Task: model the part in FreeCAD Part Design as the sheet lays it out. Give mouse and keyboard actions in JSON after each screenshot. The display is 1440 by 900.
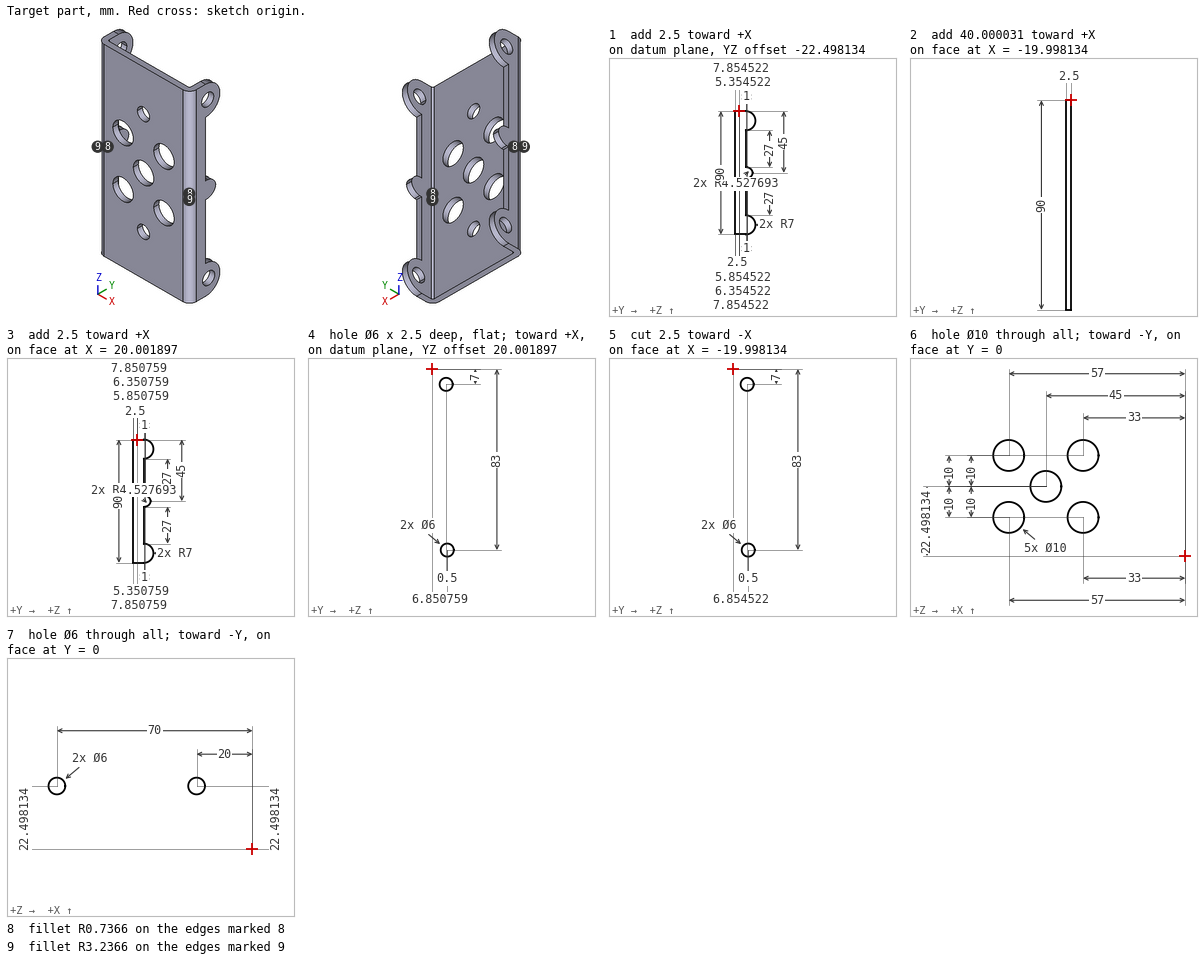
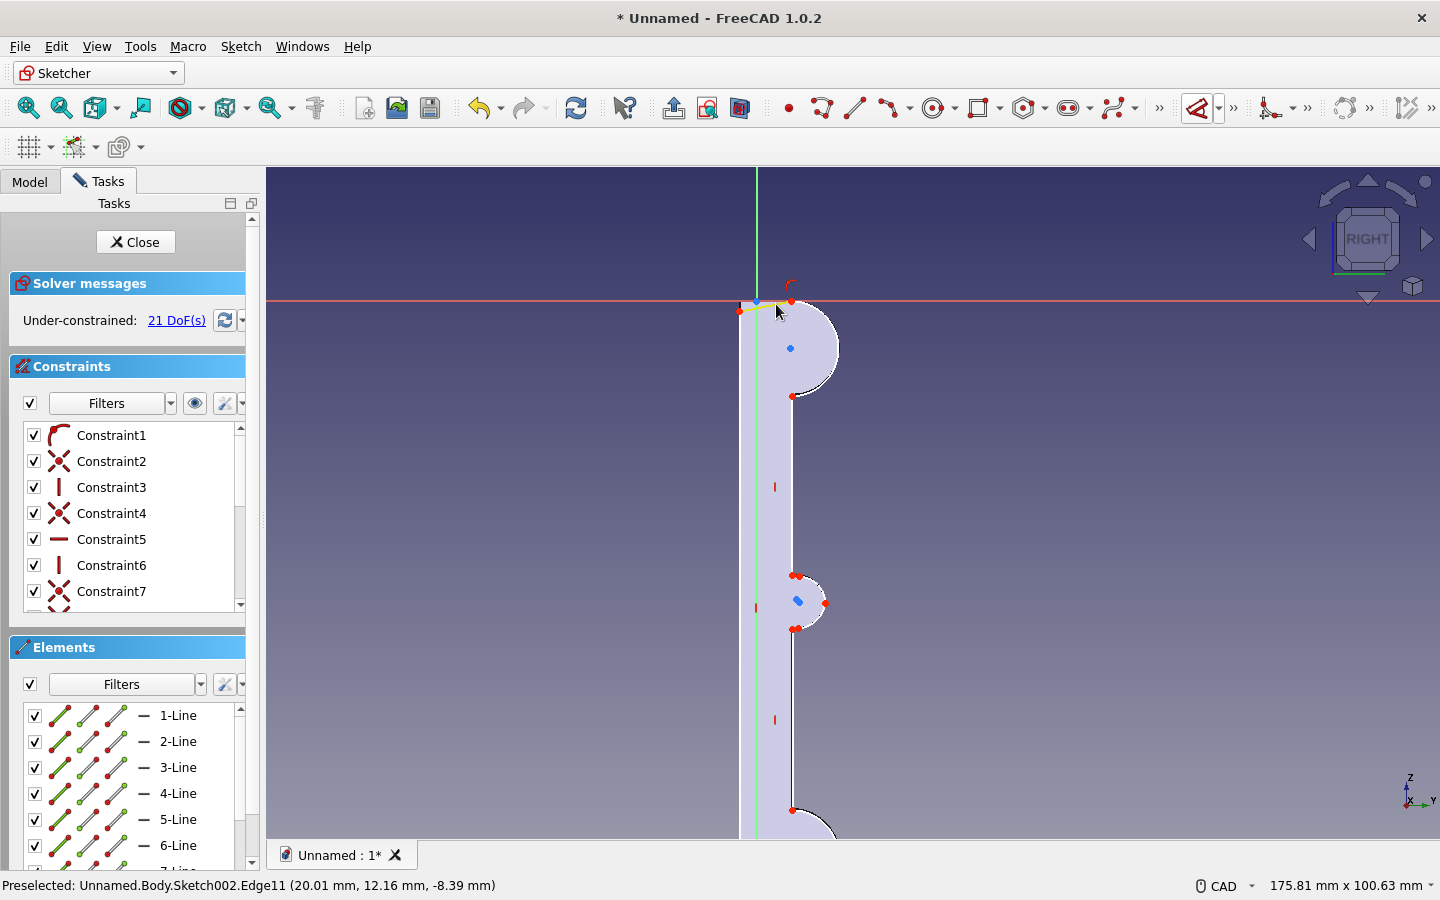
{"action": "left_click", "coordinate": [776, 304]}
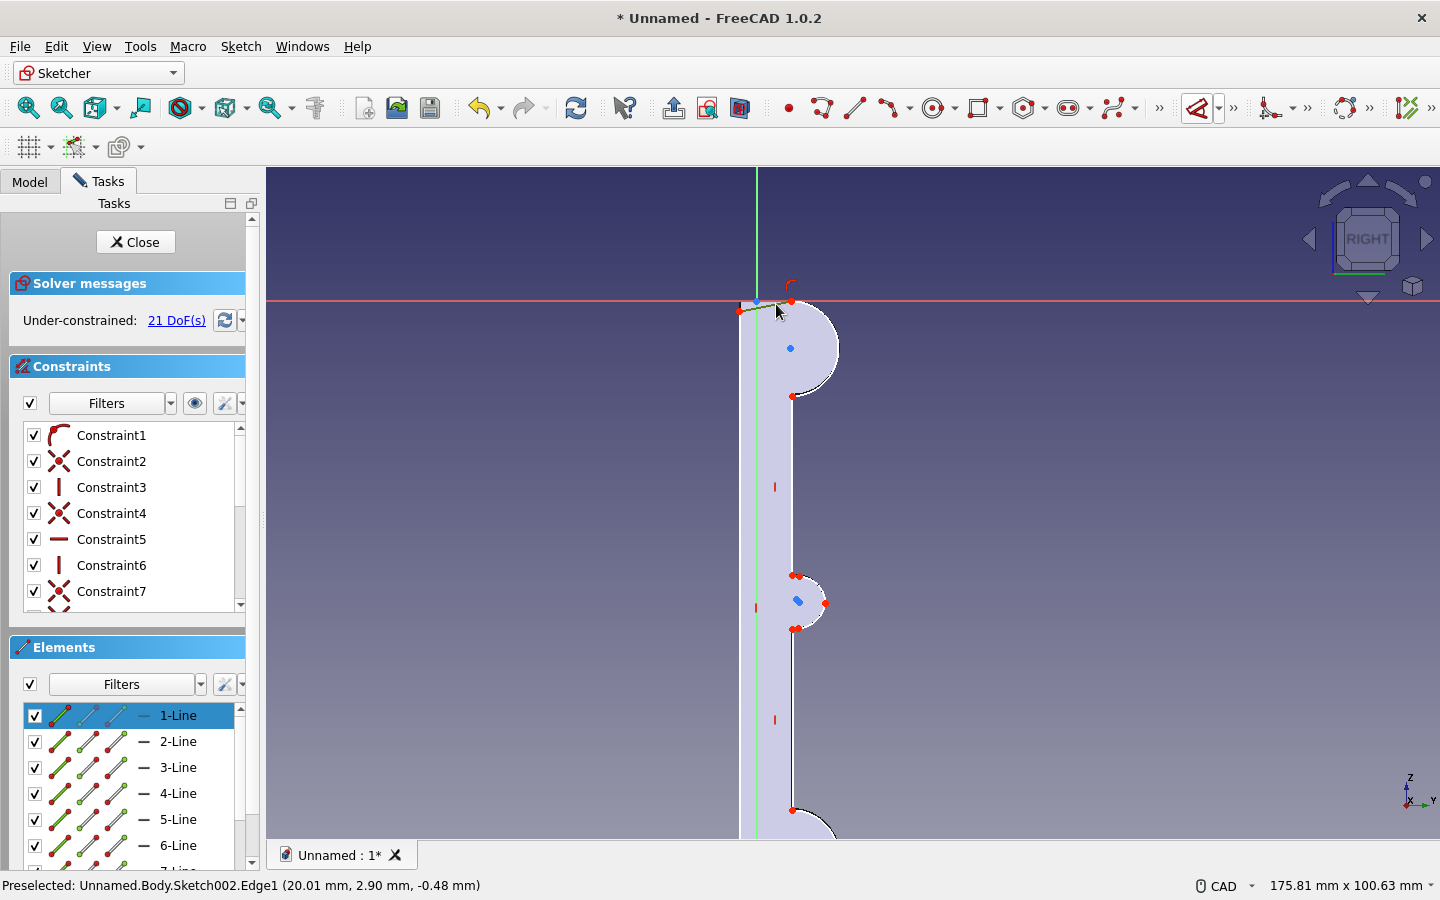
{"action": "left_click", "coordinate": [830, 376]}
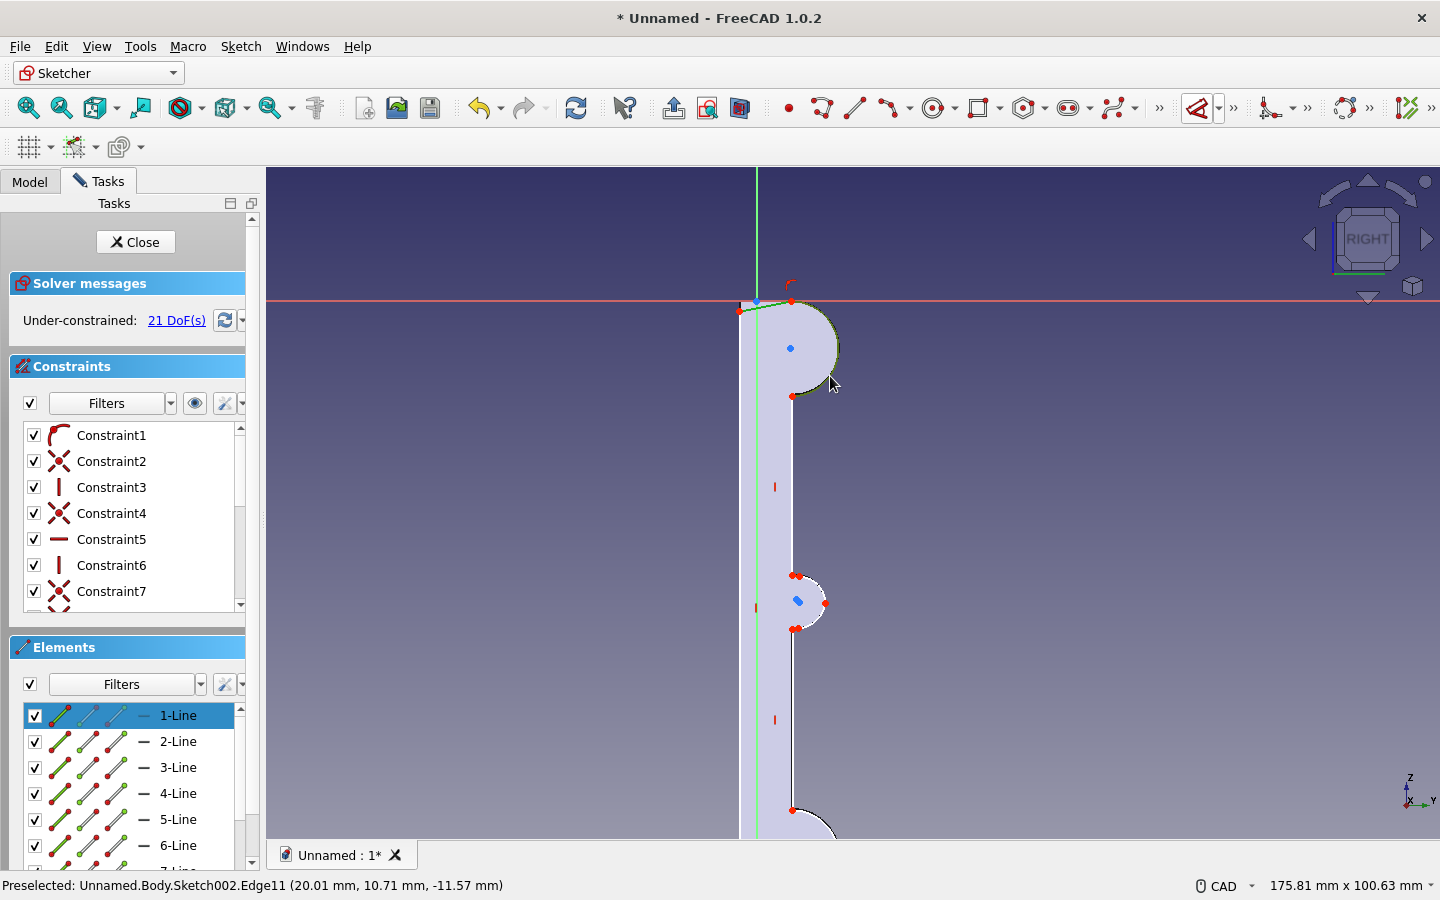
{"action": "key", "text": "t"}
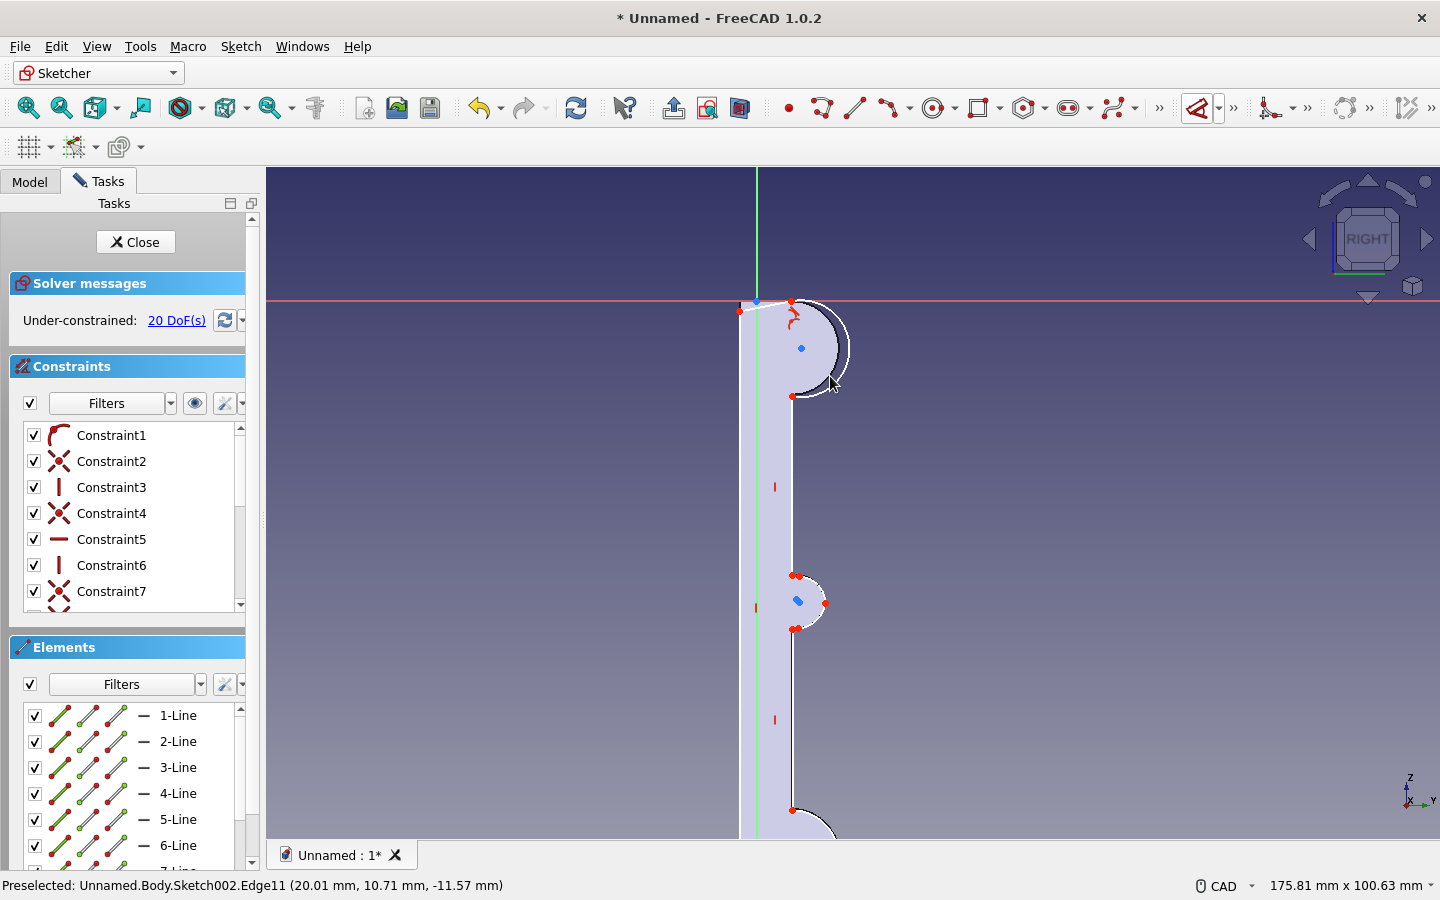
{"action": "scroll", "coordinate": [774, 302], "scroll_direction": "down", "scroll_amount": 2}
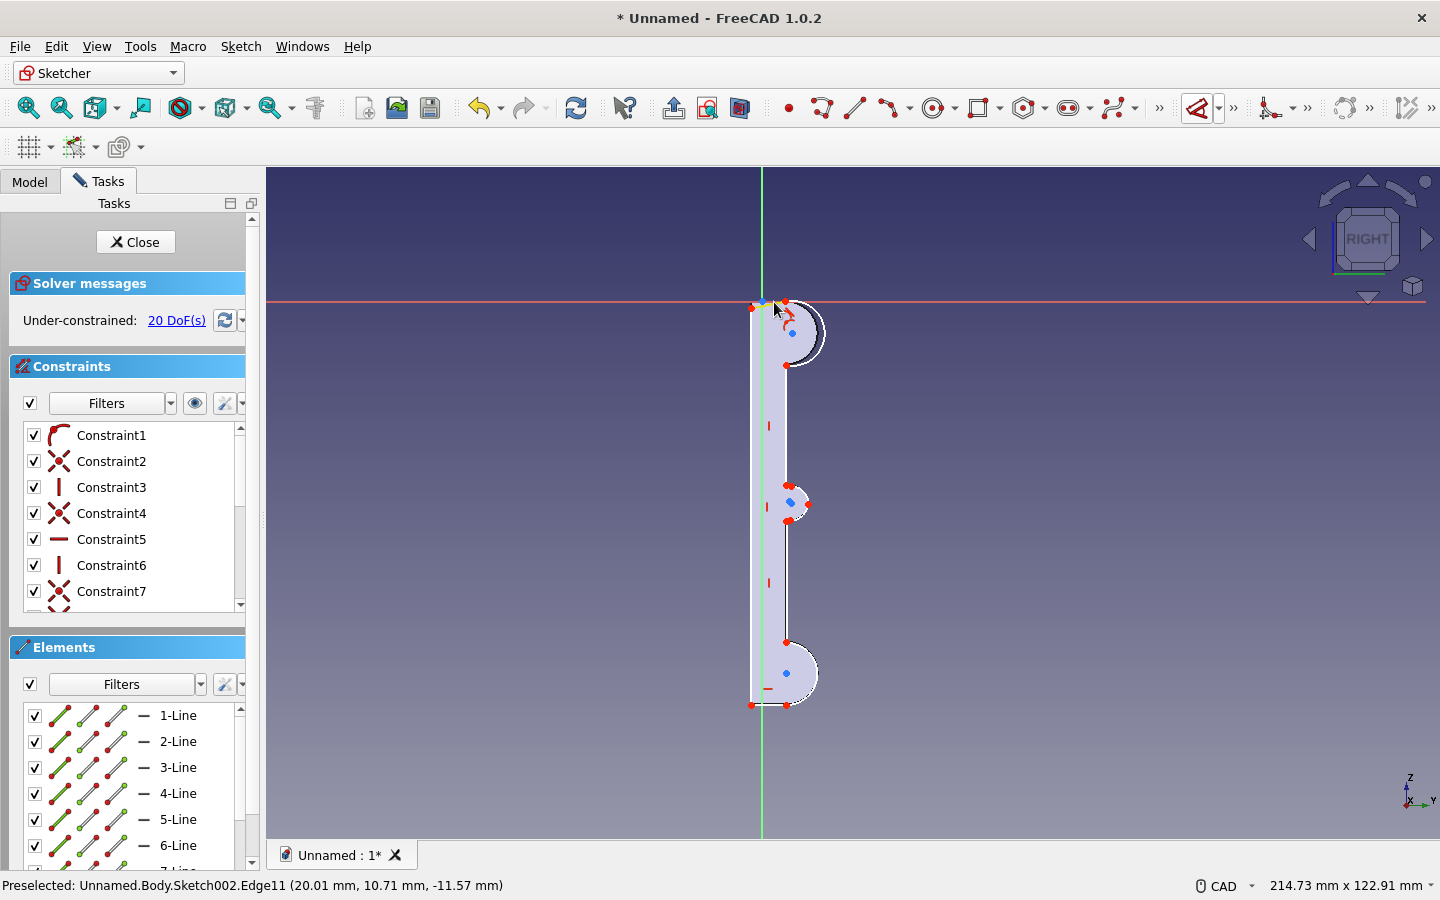
{"action": "scroll", "coordinate": [762, 705], "scroll_direction": "up", "scroll_amount": 2}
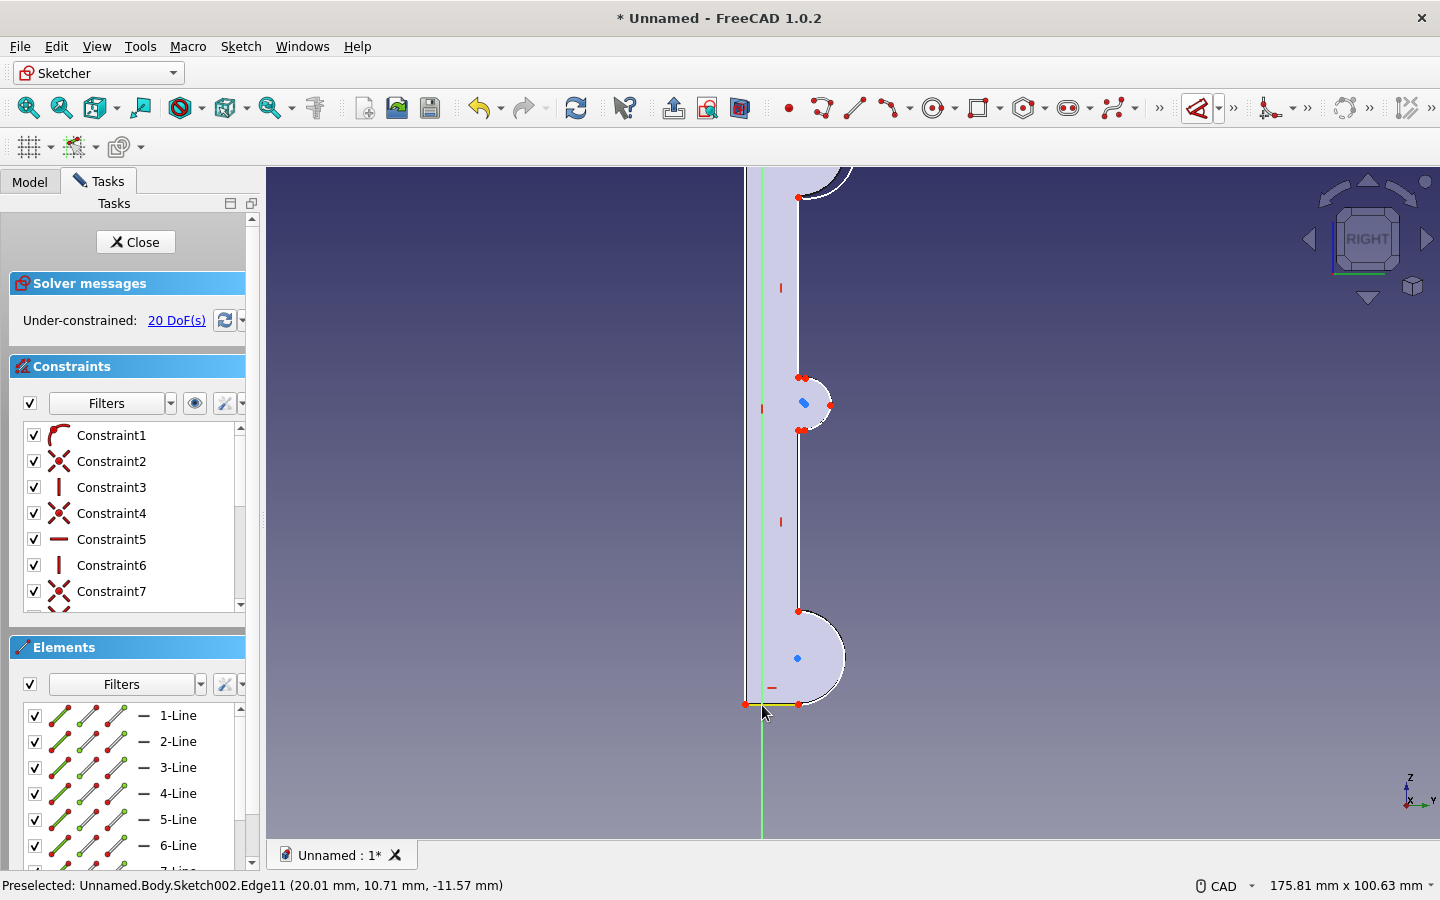
{"action": "left_click", "coordinate": [761, 705]}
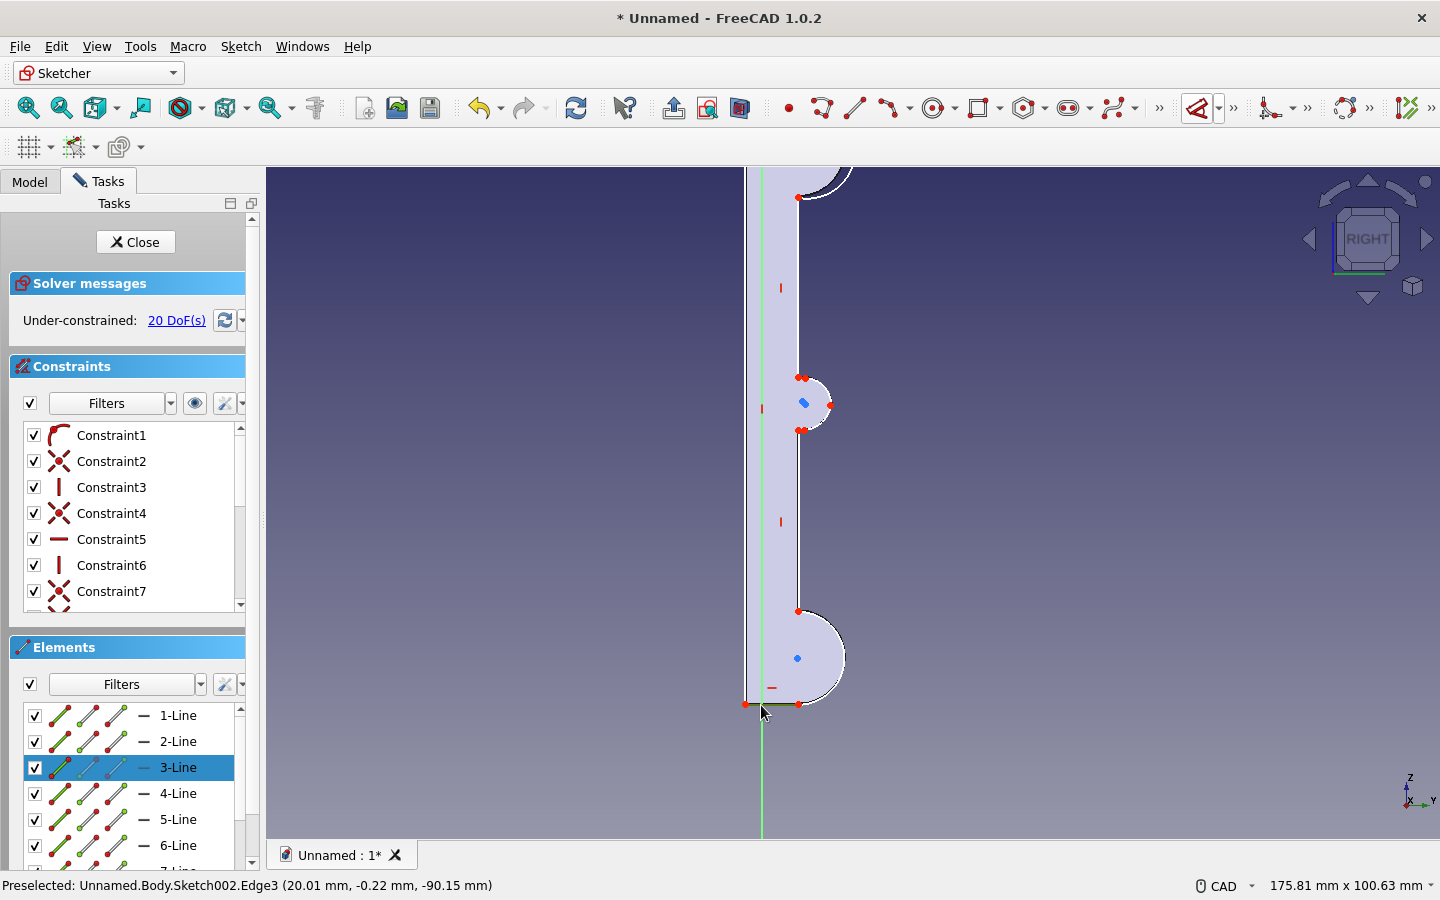
{"action": "left_click", "coordinate": [836, 685]}